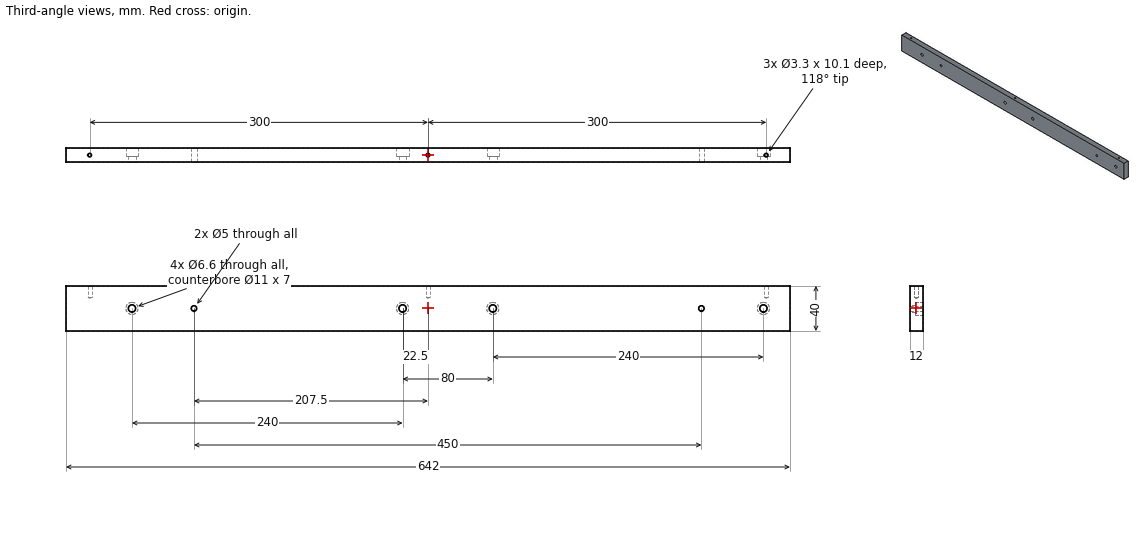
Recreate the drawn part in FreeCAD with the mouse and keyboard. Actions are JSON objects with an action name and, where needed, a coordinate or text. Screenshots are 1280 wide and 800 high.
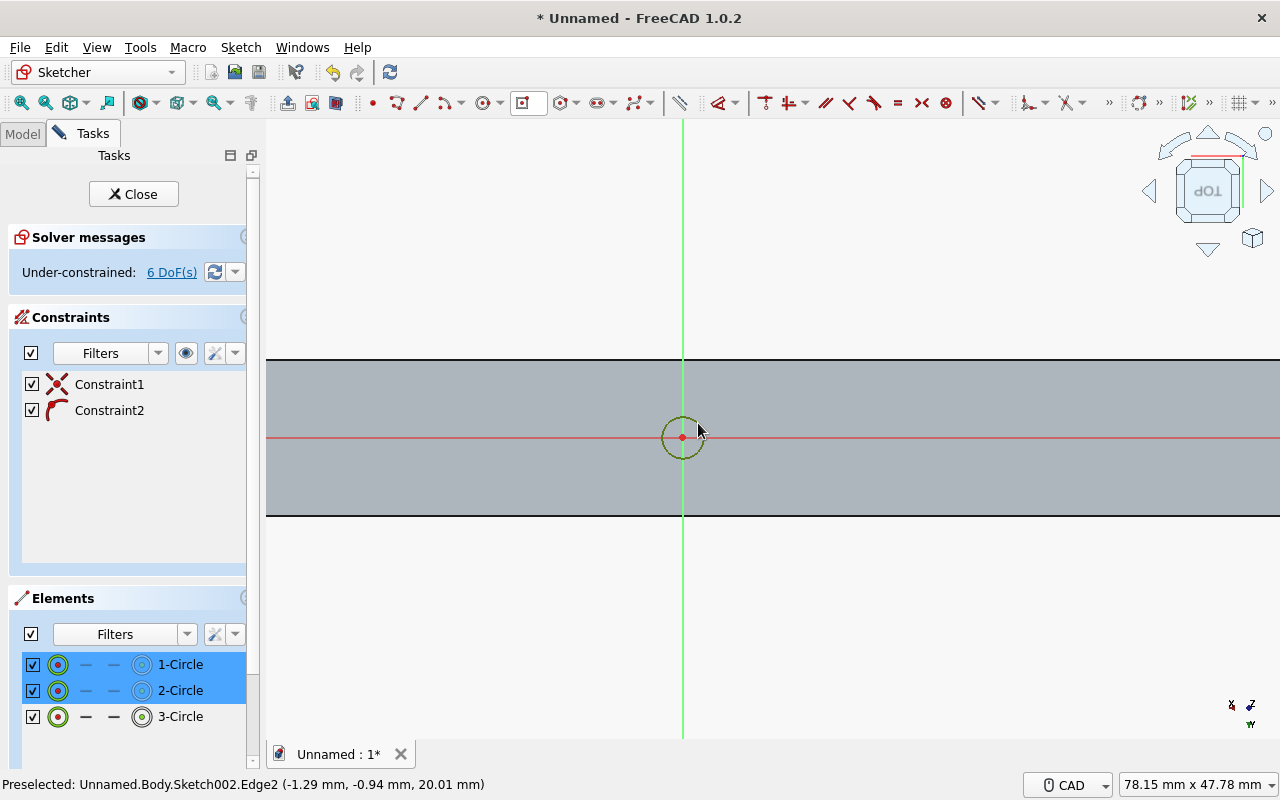
{"action": "scroll", "coordinate": [706, 428], "scroll_direction": "down", "scroll_amount": 13}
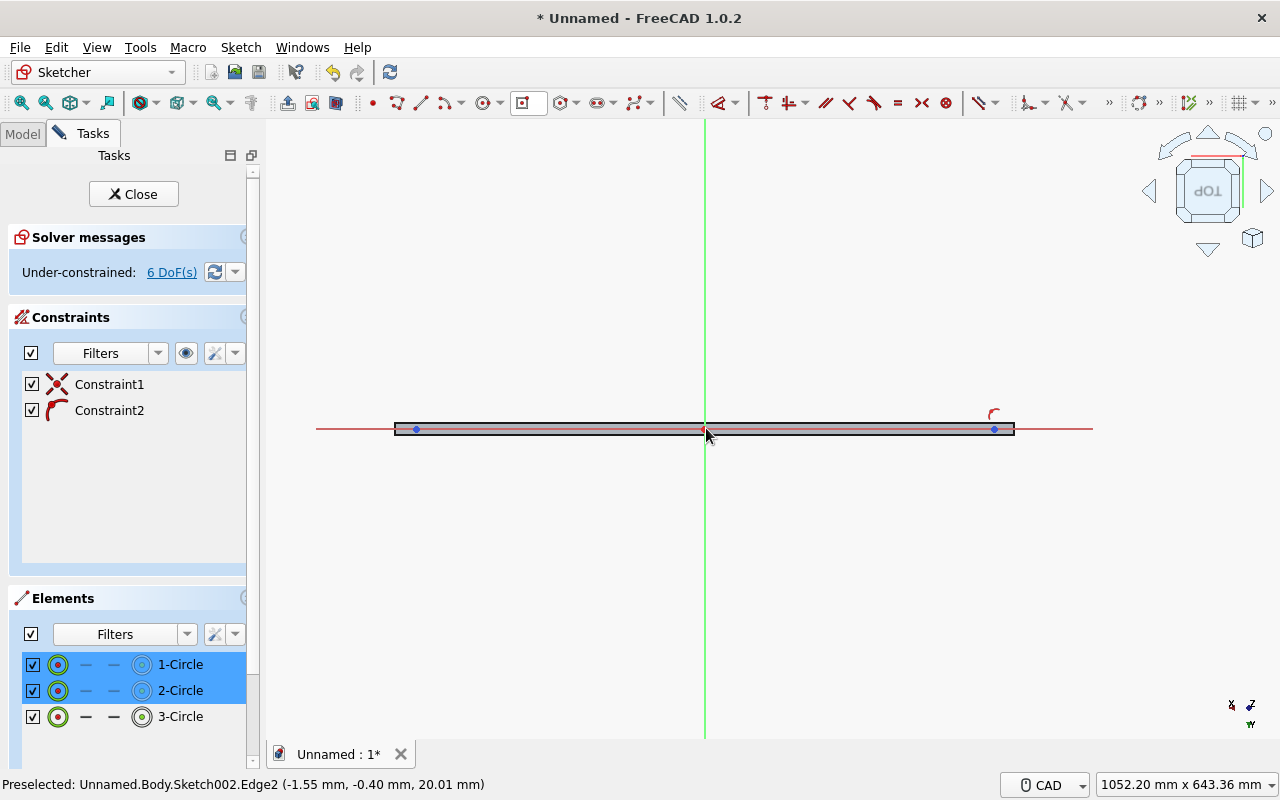
{"action": "scroll", "coordinate": [995, 428], "scroll_direction": "up", "scroll_amount": 12}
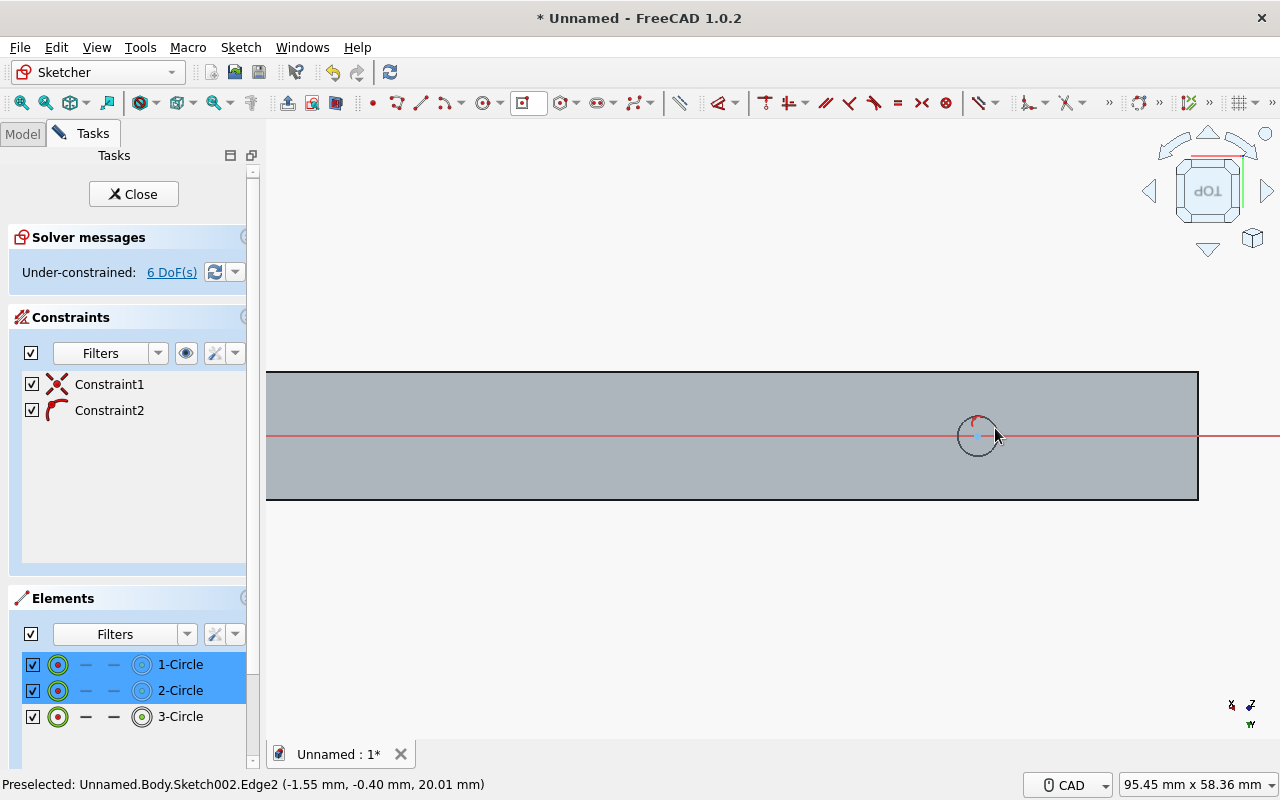
{"action": "left_click", "coordinate": [992, 422]}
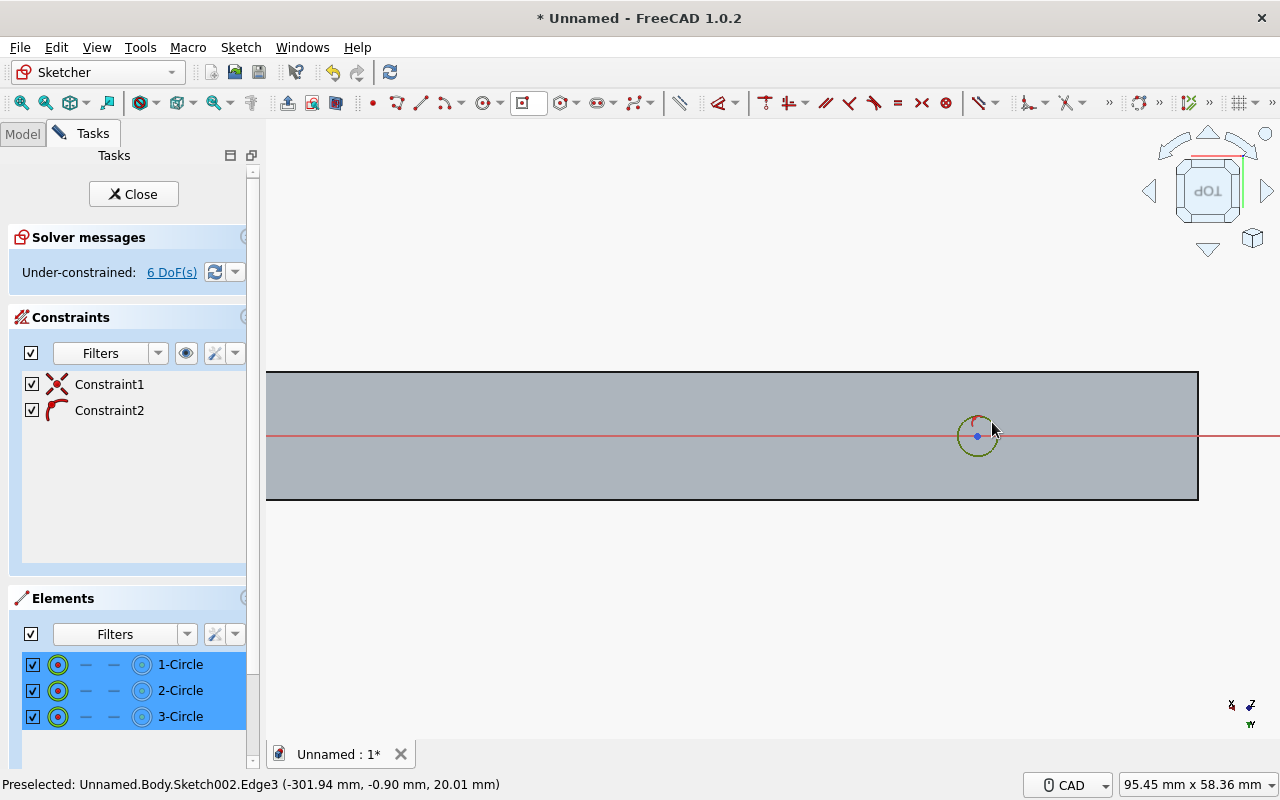
{"action": "left_click", "coordinate": [898, 104]}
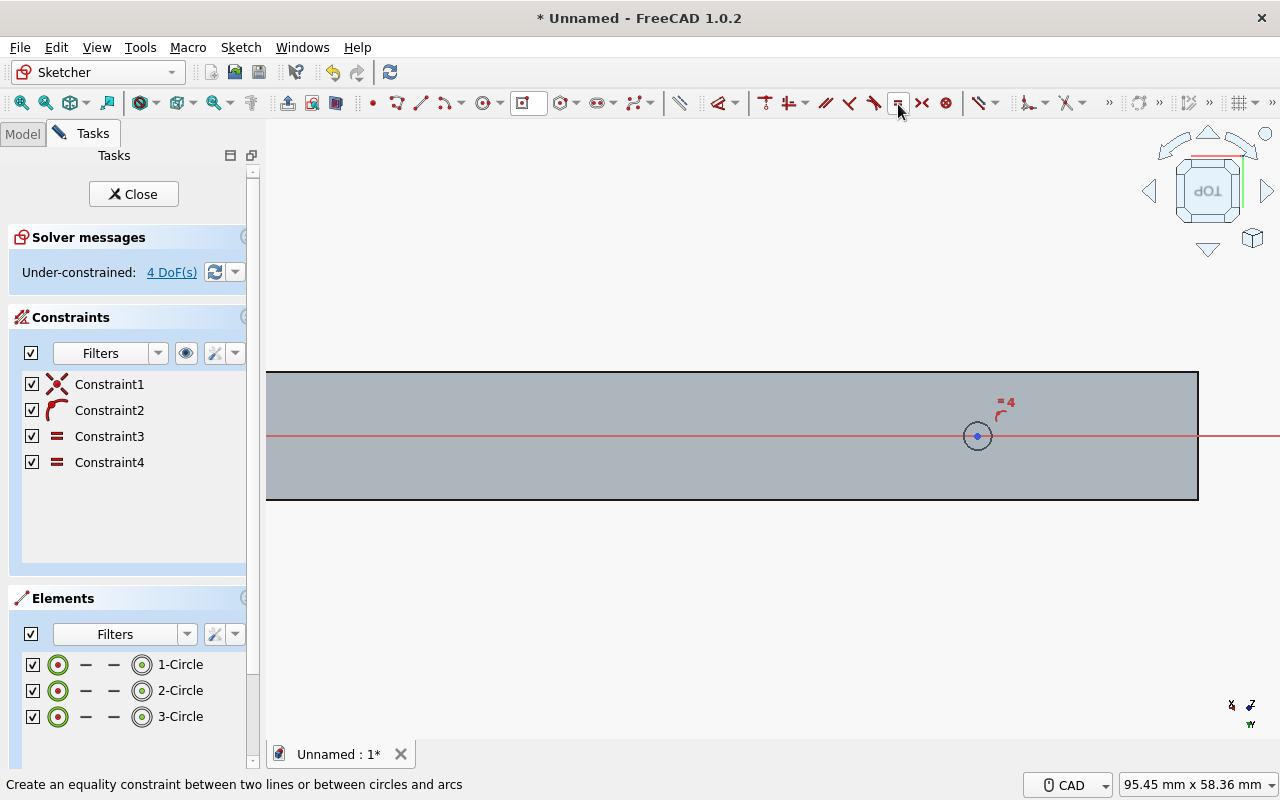
{"action": "scroll", "coordinate": [996, 428], "scroll_direction": "down", "scroll_amount": 12}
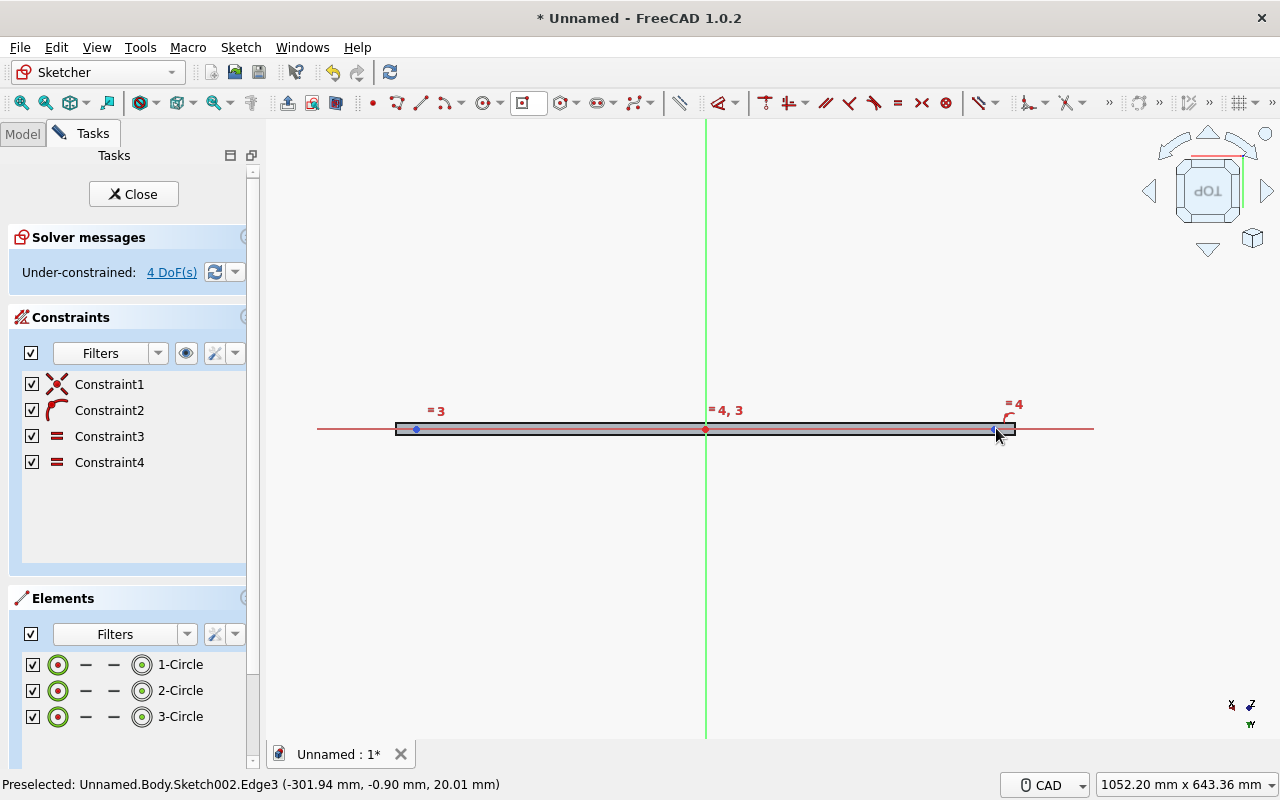
{"action": "left_click", "coordinate": [417, 430]}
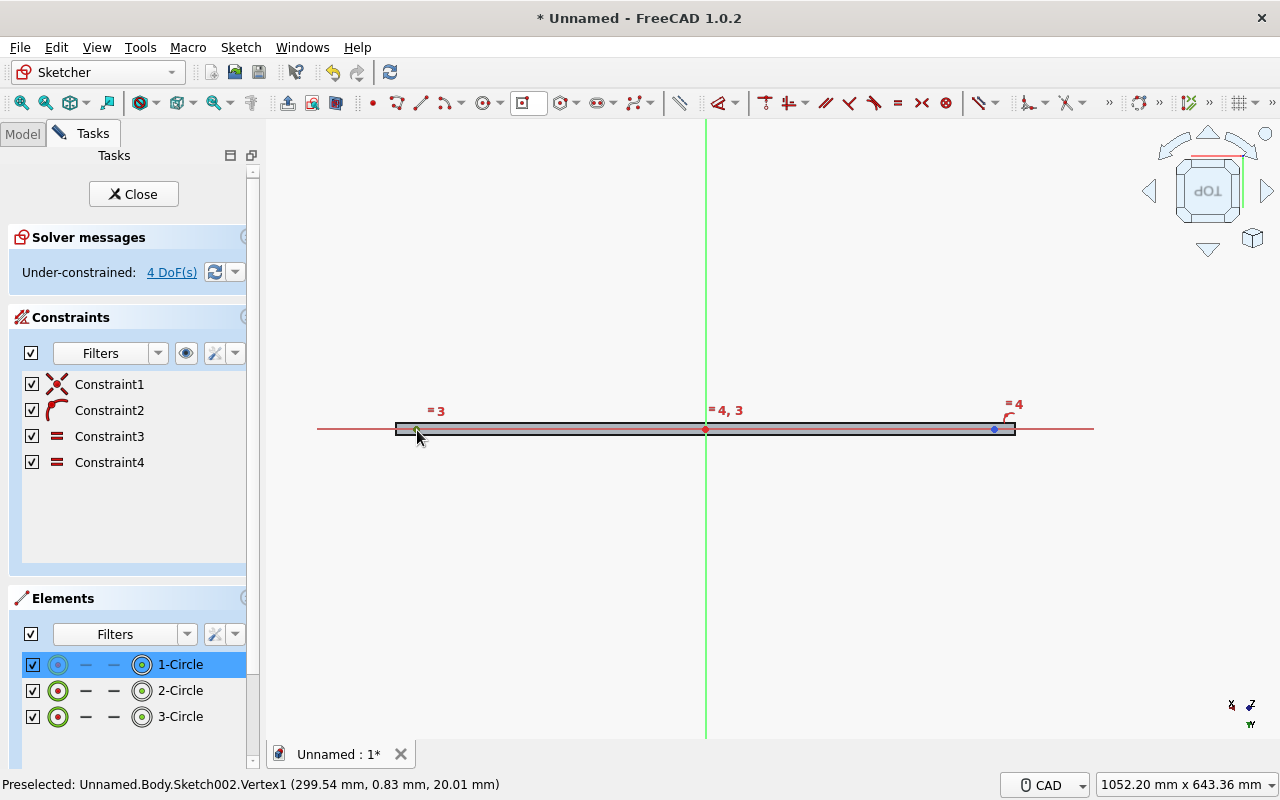
{"action": "left_click", "coordinate": [353, 429]}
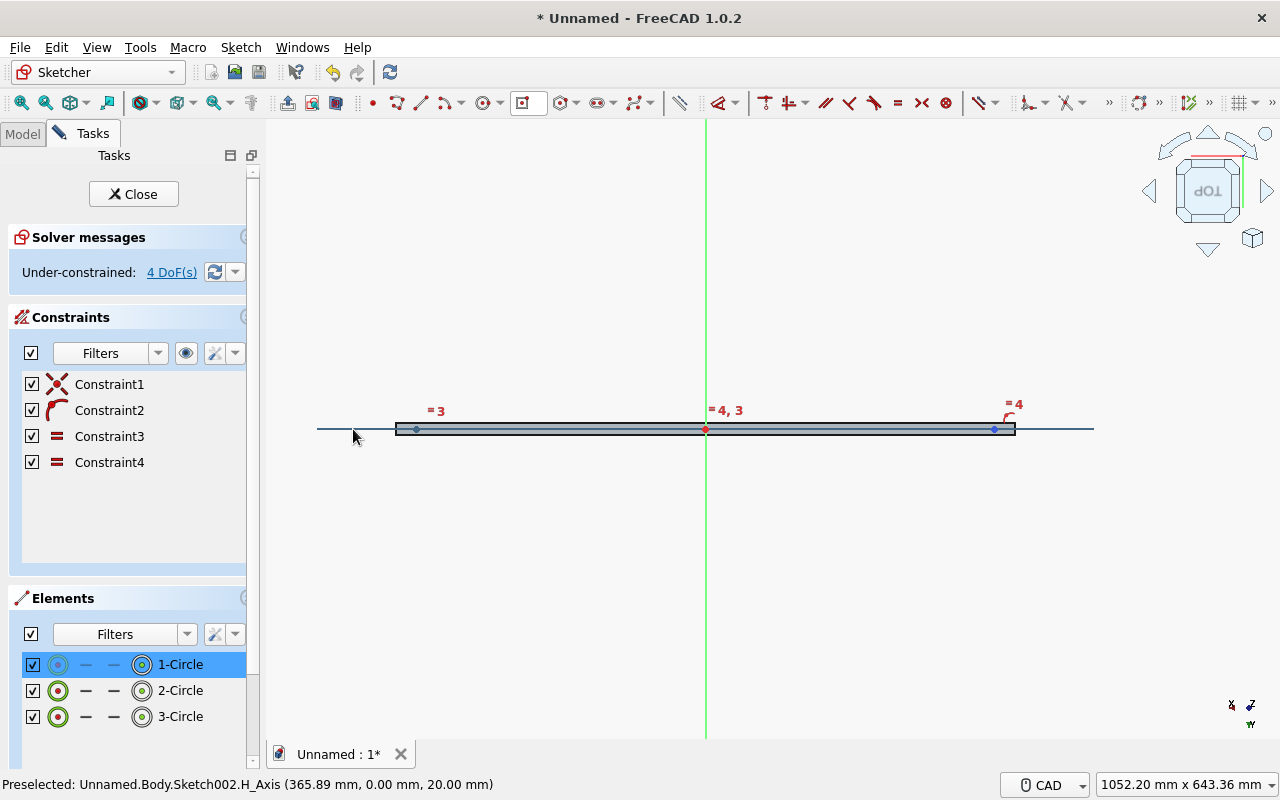
{"action": "left_click", "coordinate": [766, 104]}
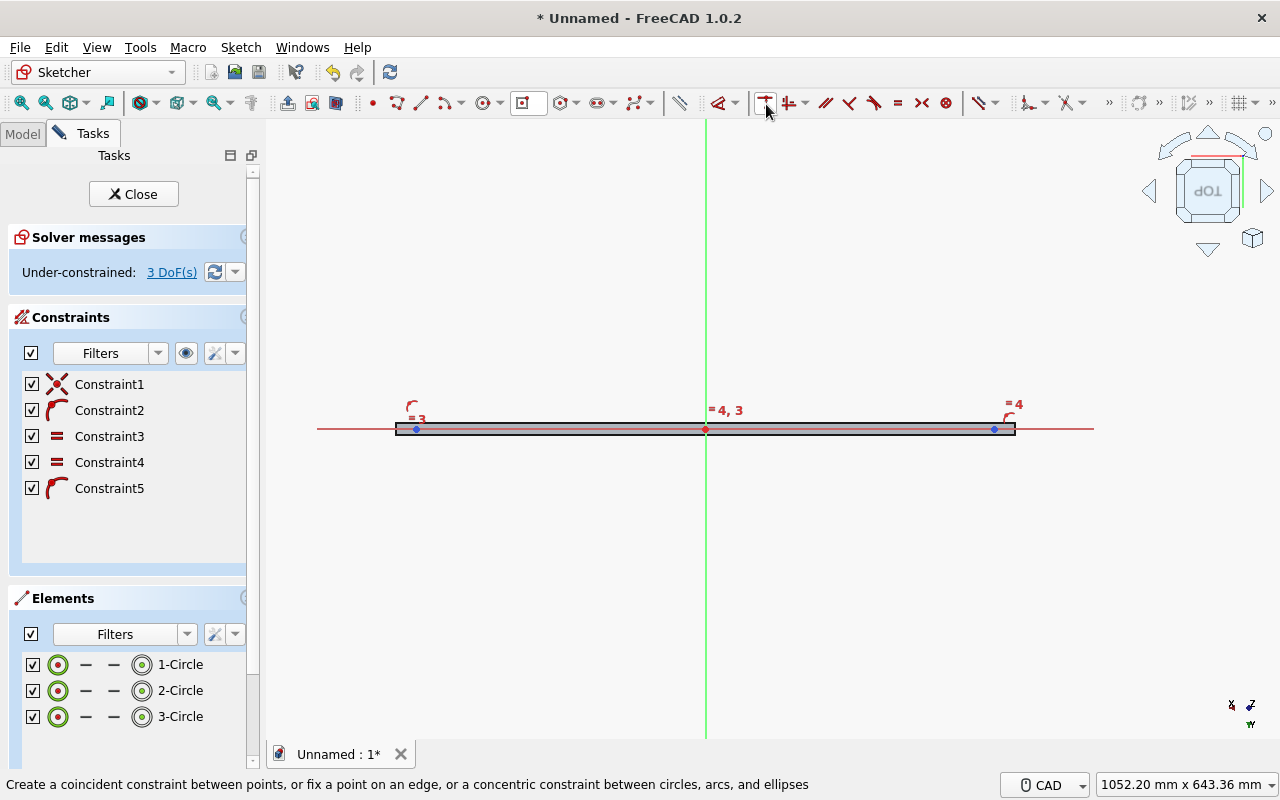
{"action": "left_click", "coordinate": [718, 104]}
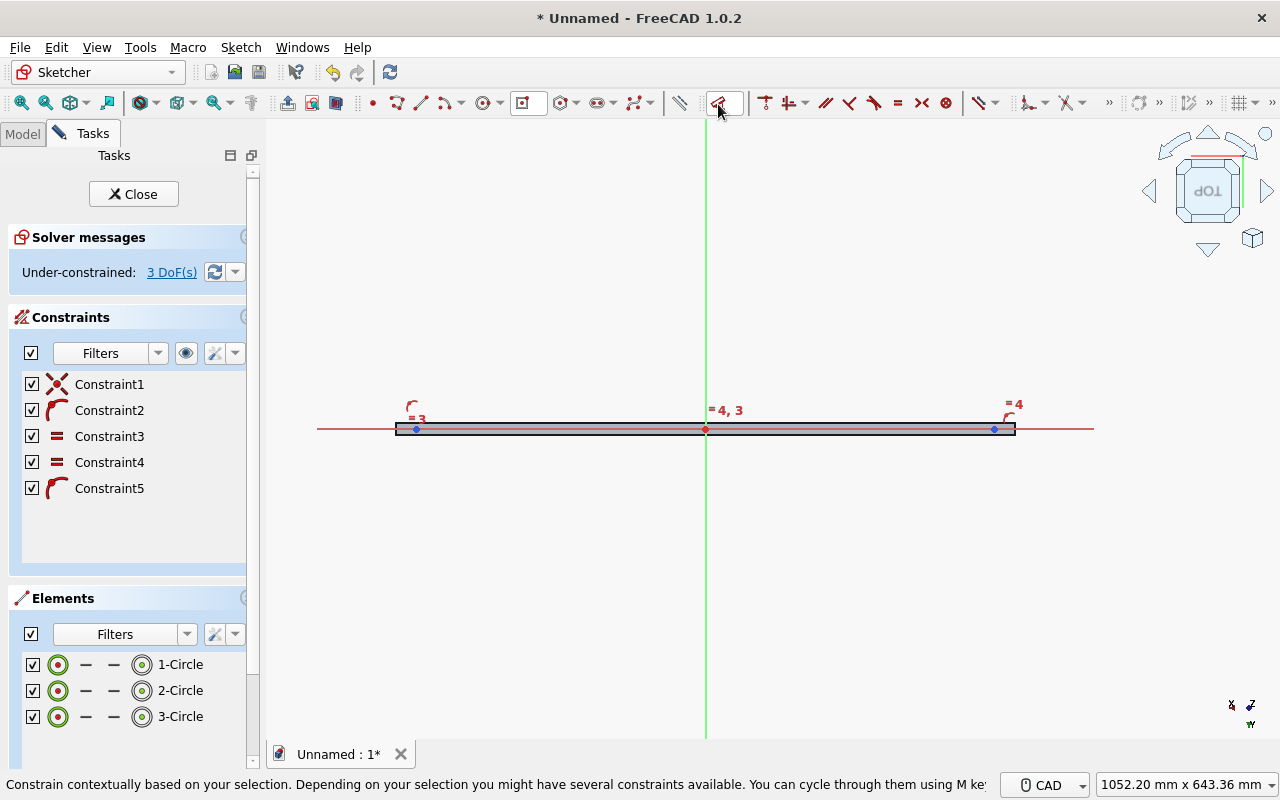
{"action": "scroll", "coordinate": [416, 429], "scroll_direction": "up", "scroll_amount": 13}